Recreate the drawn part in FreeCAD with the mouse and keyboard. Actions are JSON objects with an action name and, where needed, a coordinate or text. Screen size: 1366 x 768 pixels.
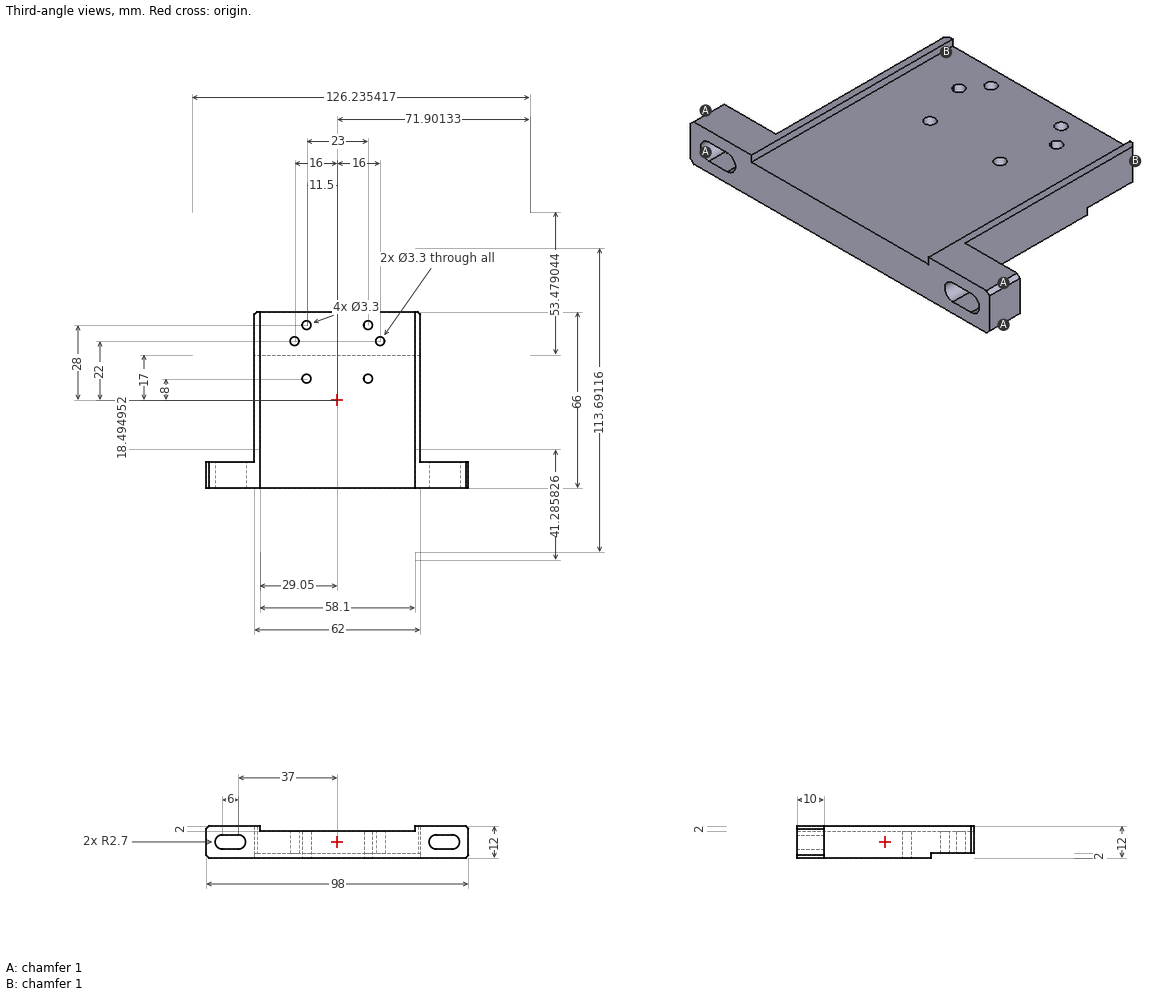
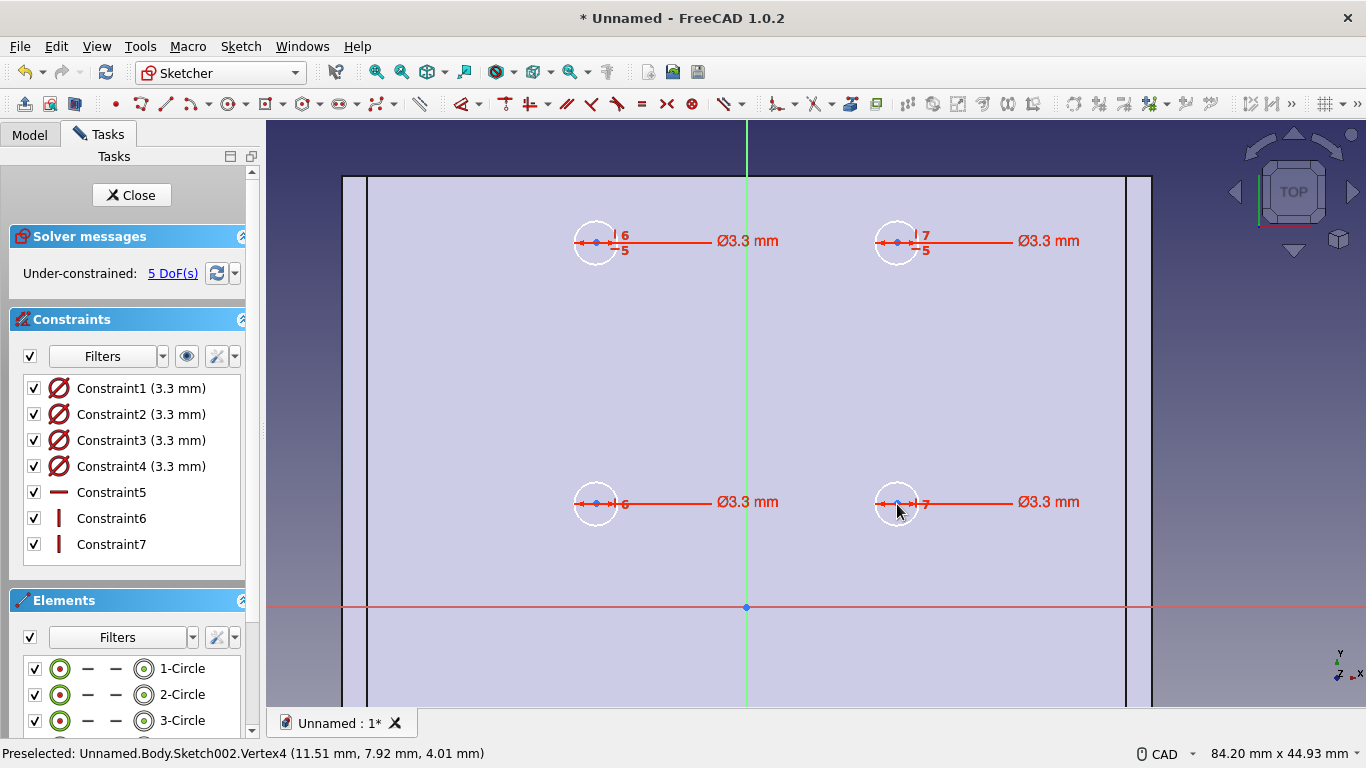
{"action": "left_click", "coordinate": [596, 504]}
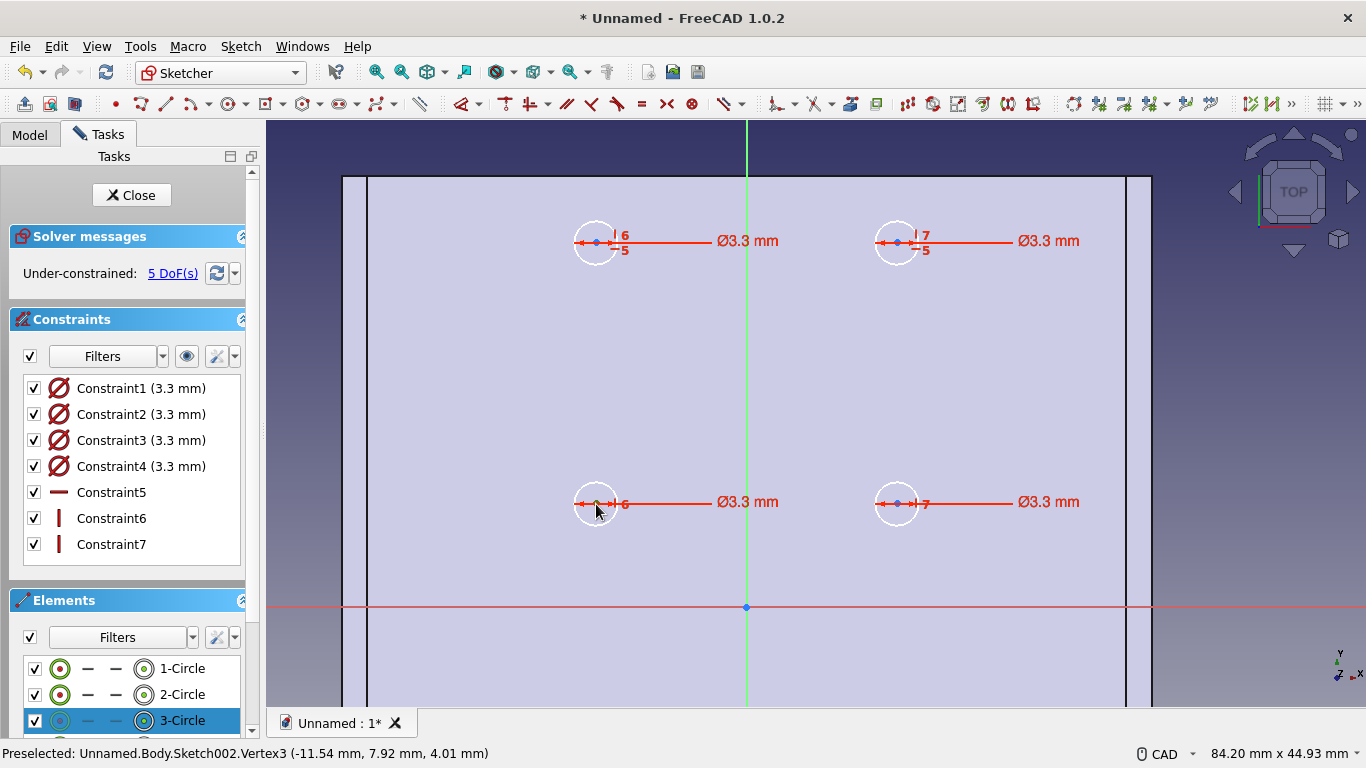
{"action": "left_click", "coordinate": [897, 504]}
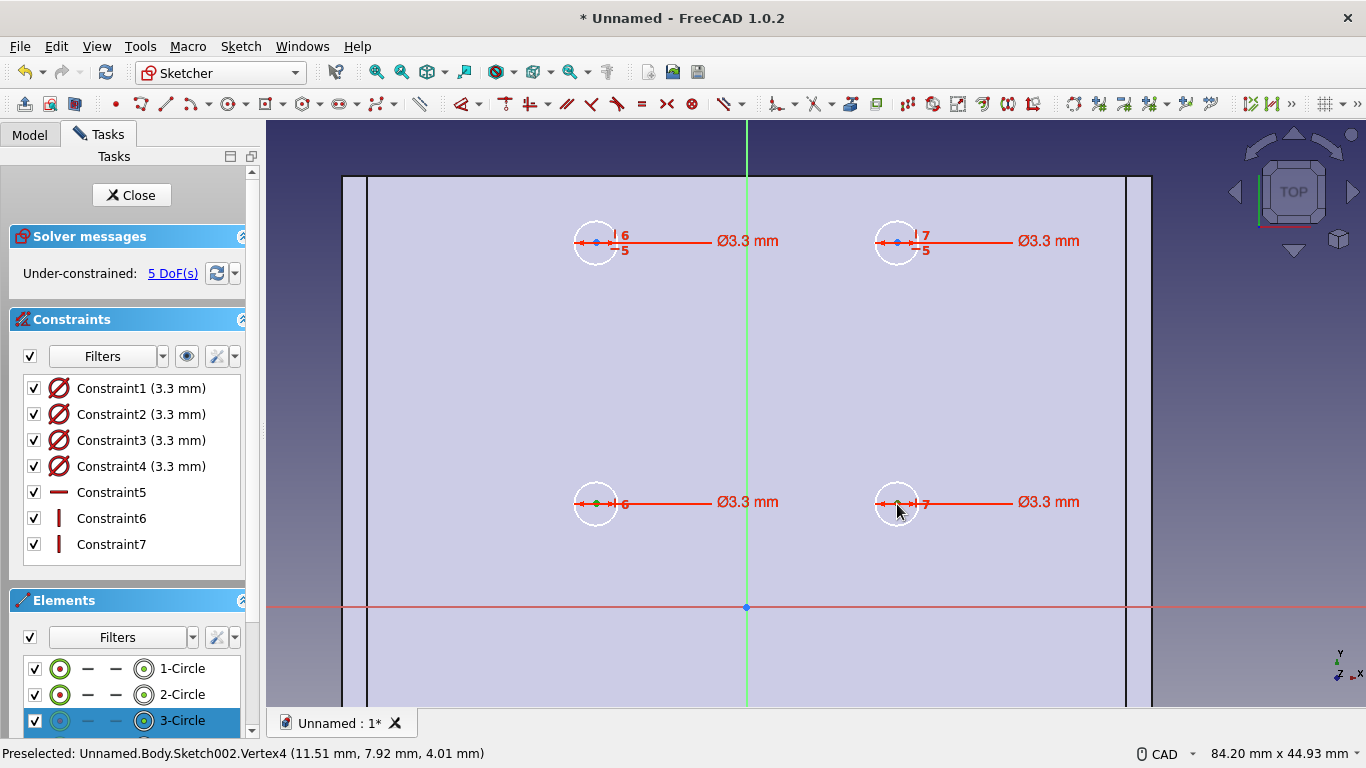
{"action": "left_click", "coordinate": [548, 104]}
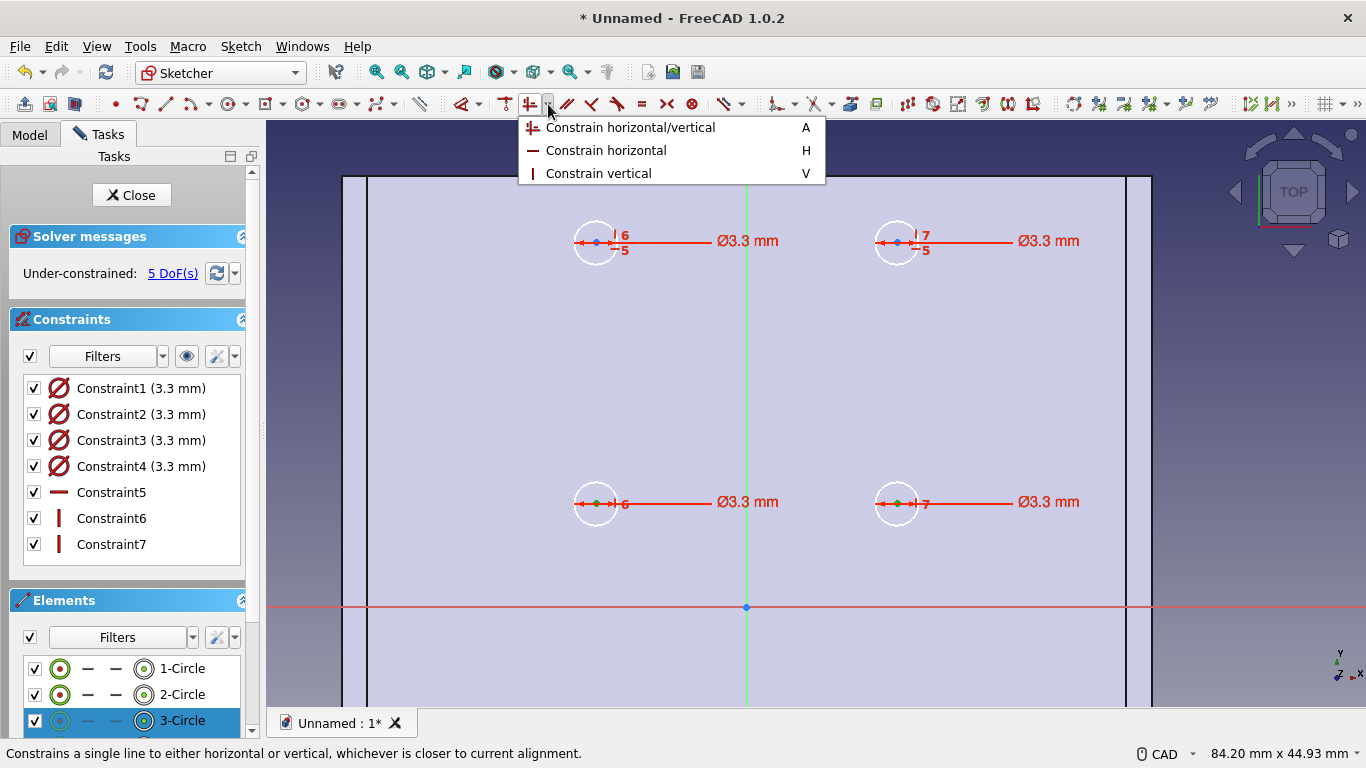
{"action": "left_click", "coordinate": [672, 150]}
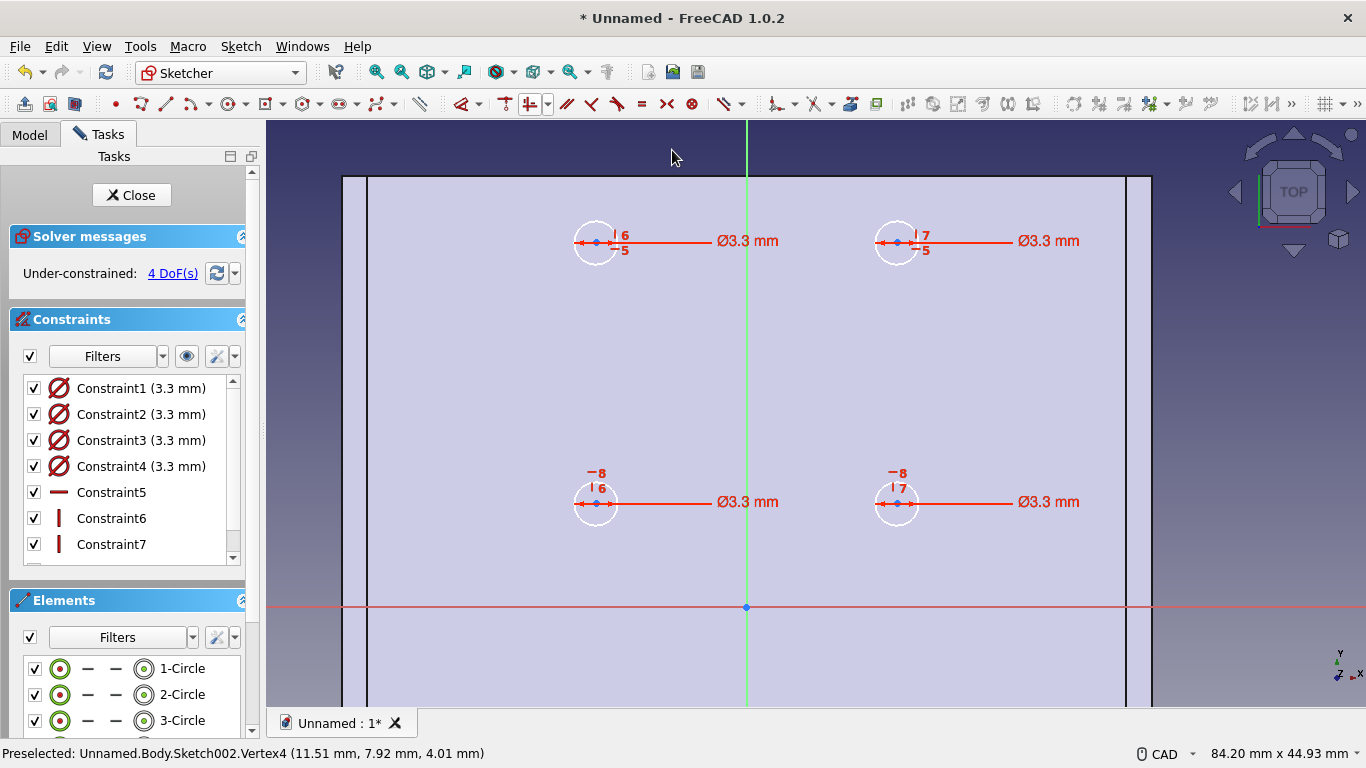
{"action": "left_click", "coordinate": [596, 504]}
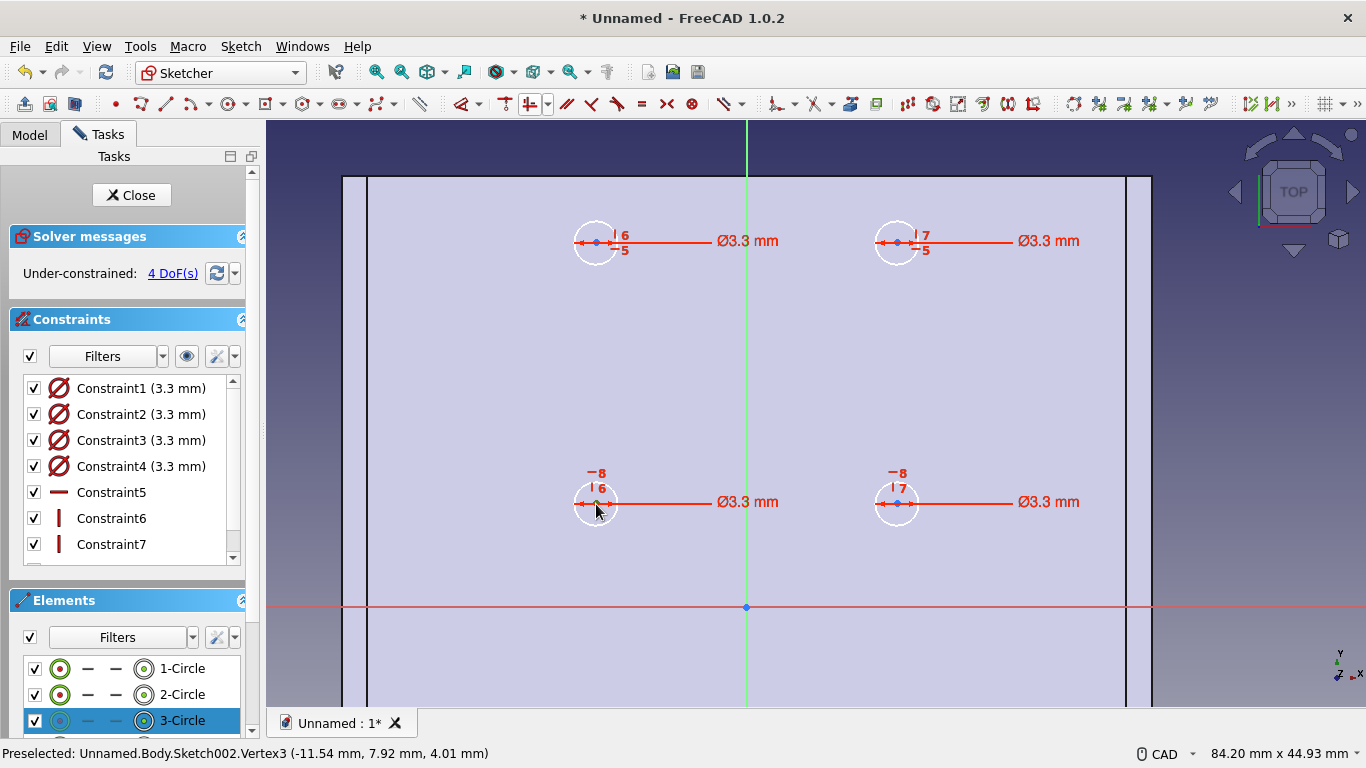
{"action": "key", "text": "i"}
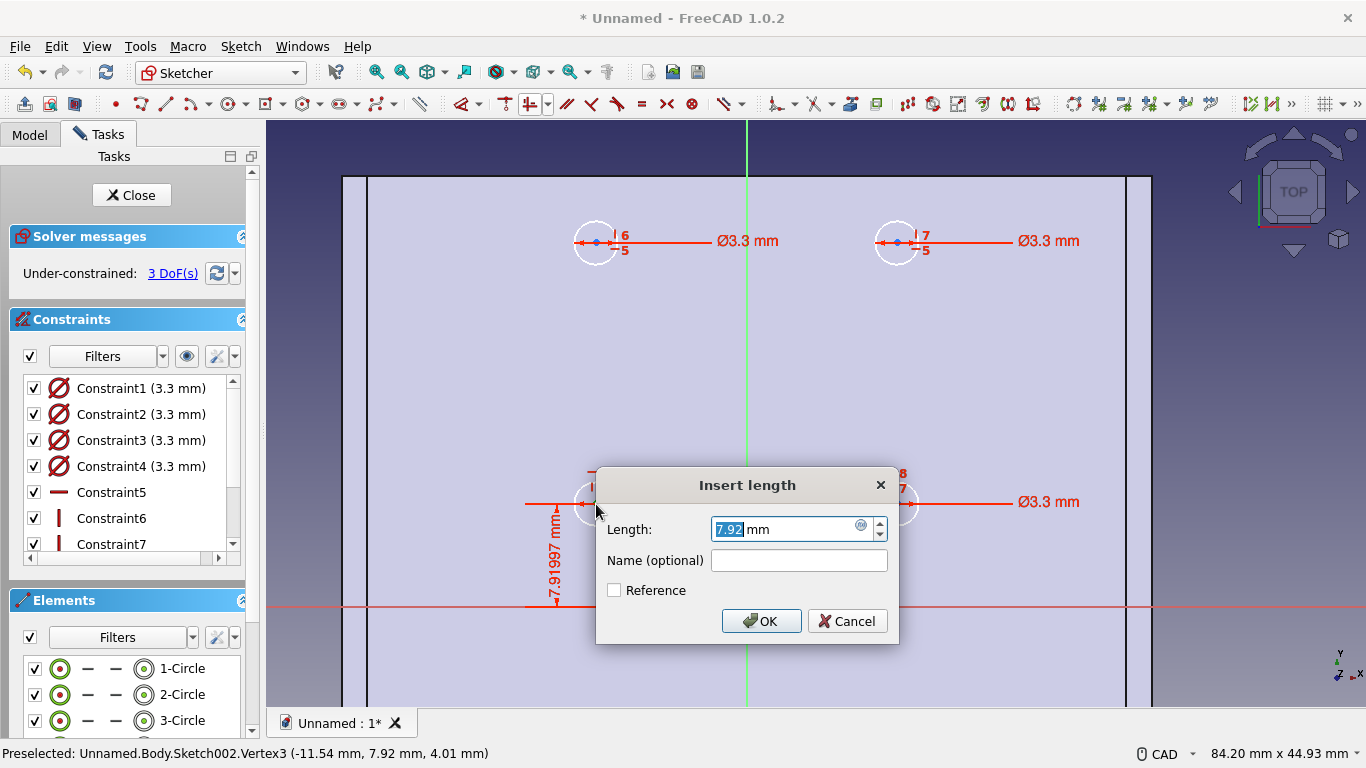
{"action": "type", "text": "8"}
{"action": "key", "text": "Return"}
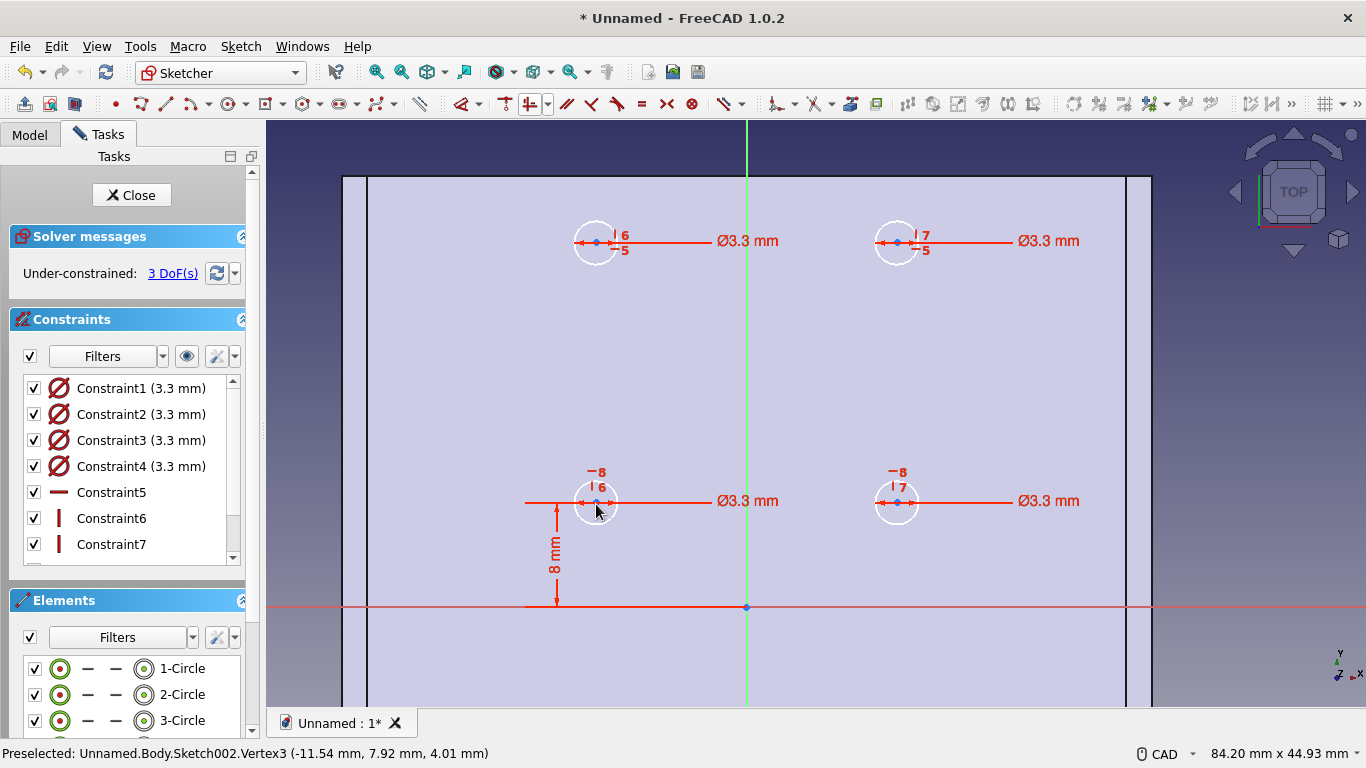
{"action": "left_click", "coordinate": [596, 243]}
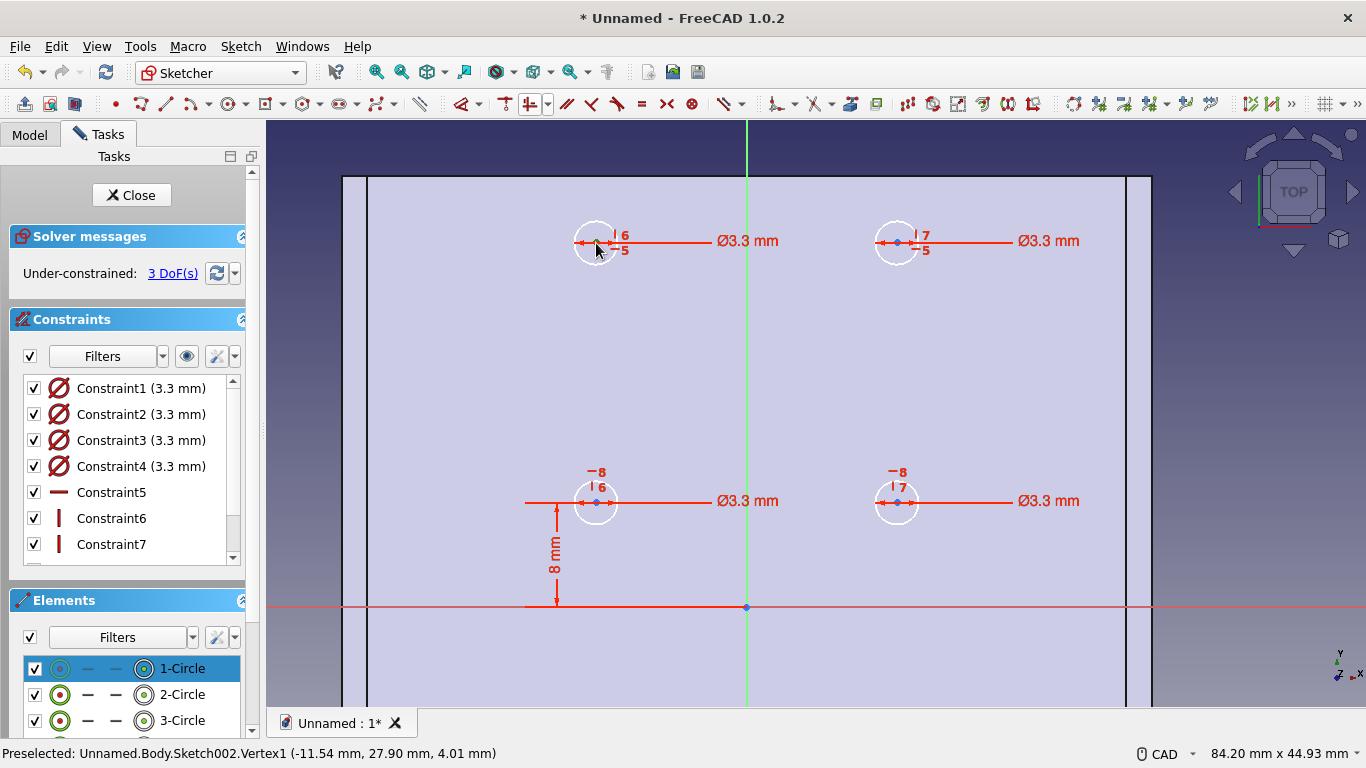
{"action": "left_click", "coordinate": [478, 104]}